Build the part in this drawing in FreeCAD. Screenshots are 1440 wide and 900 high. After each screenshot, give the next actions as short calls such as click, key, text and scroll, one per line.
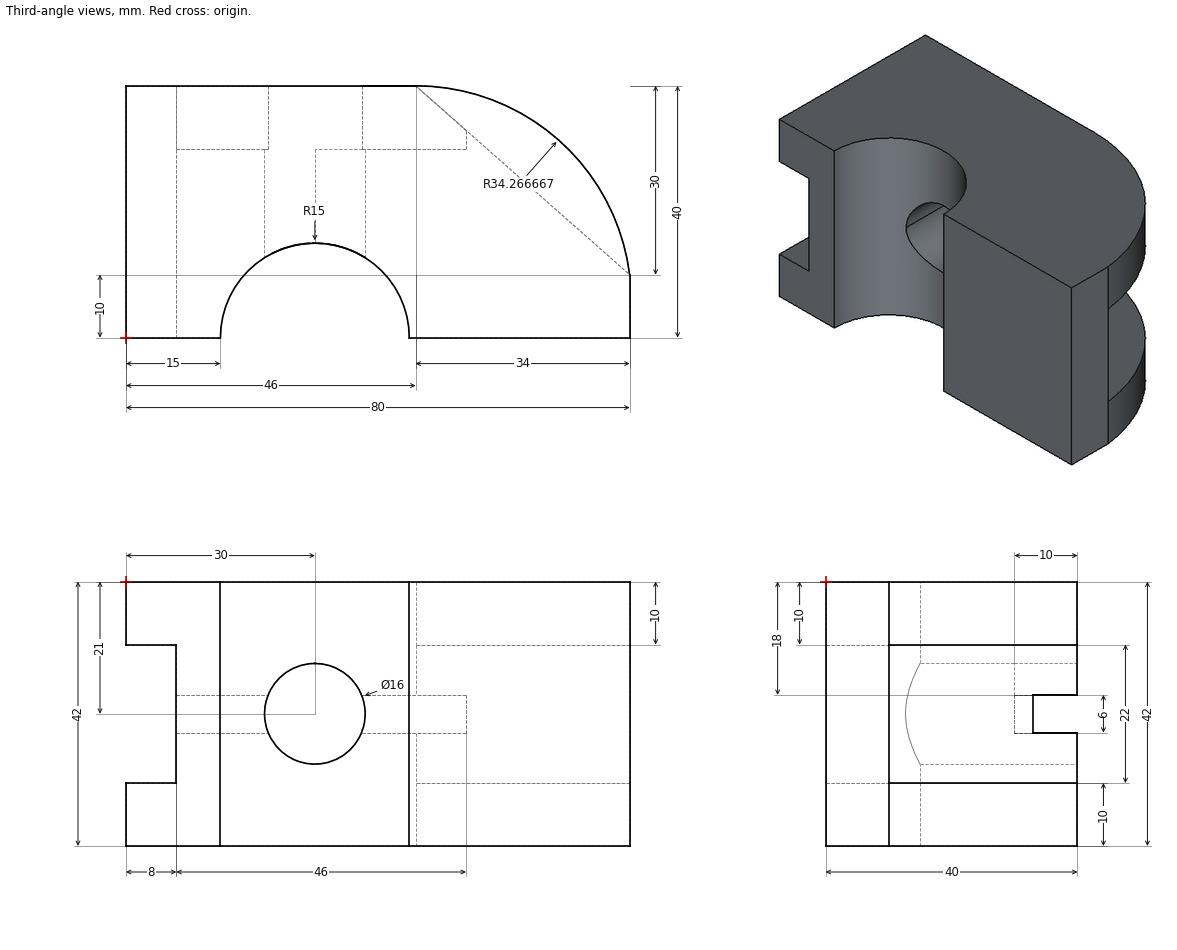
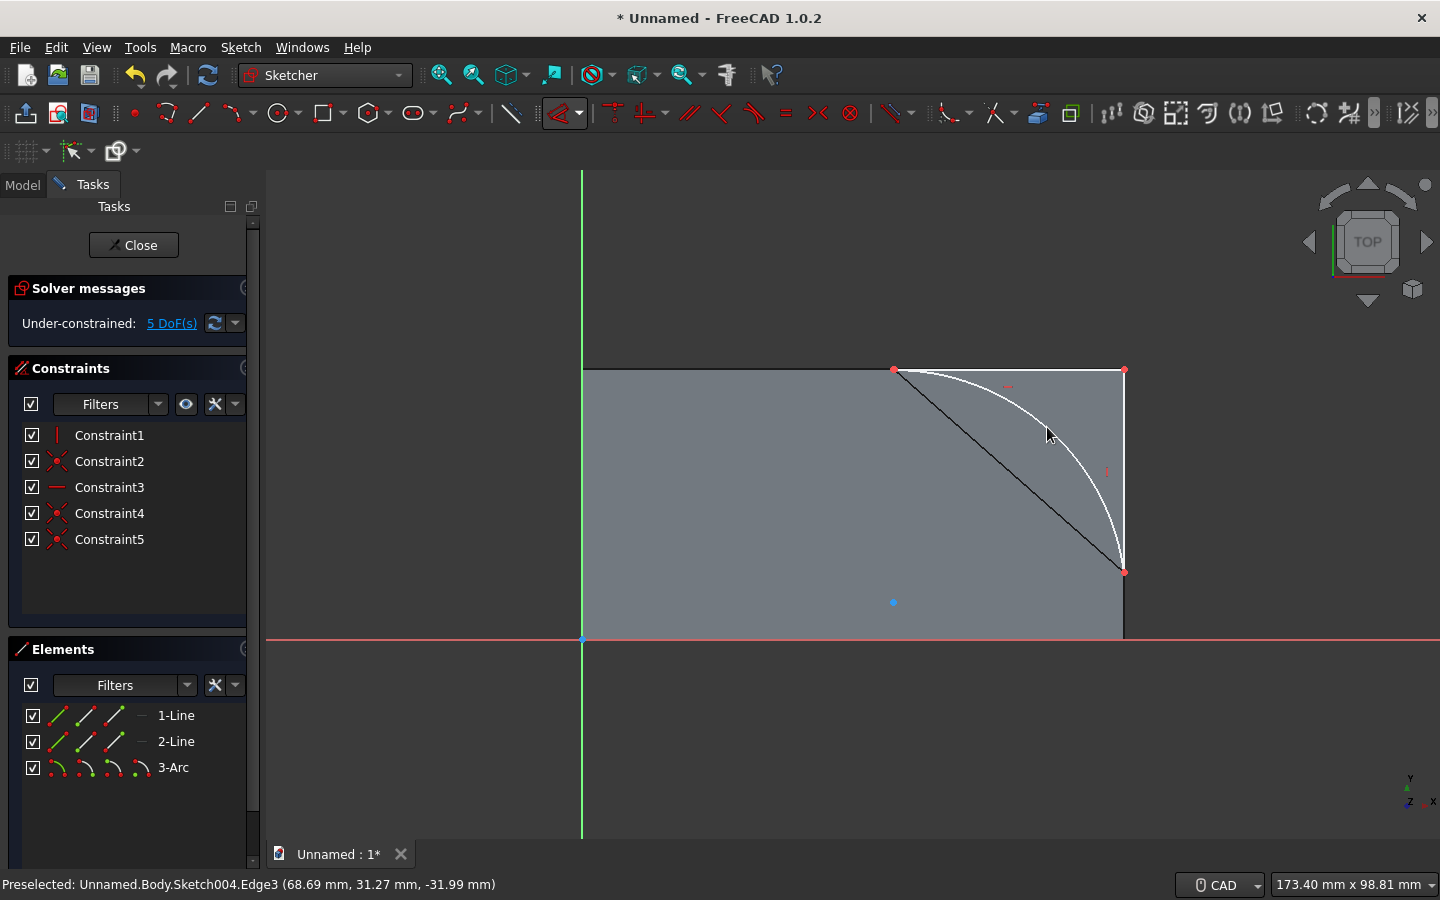
click(1055, 370)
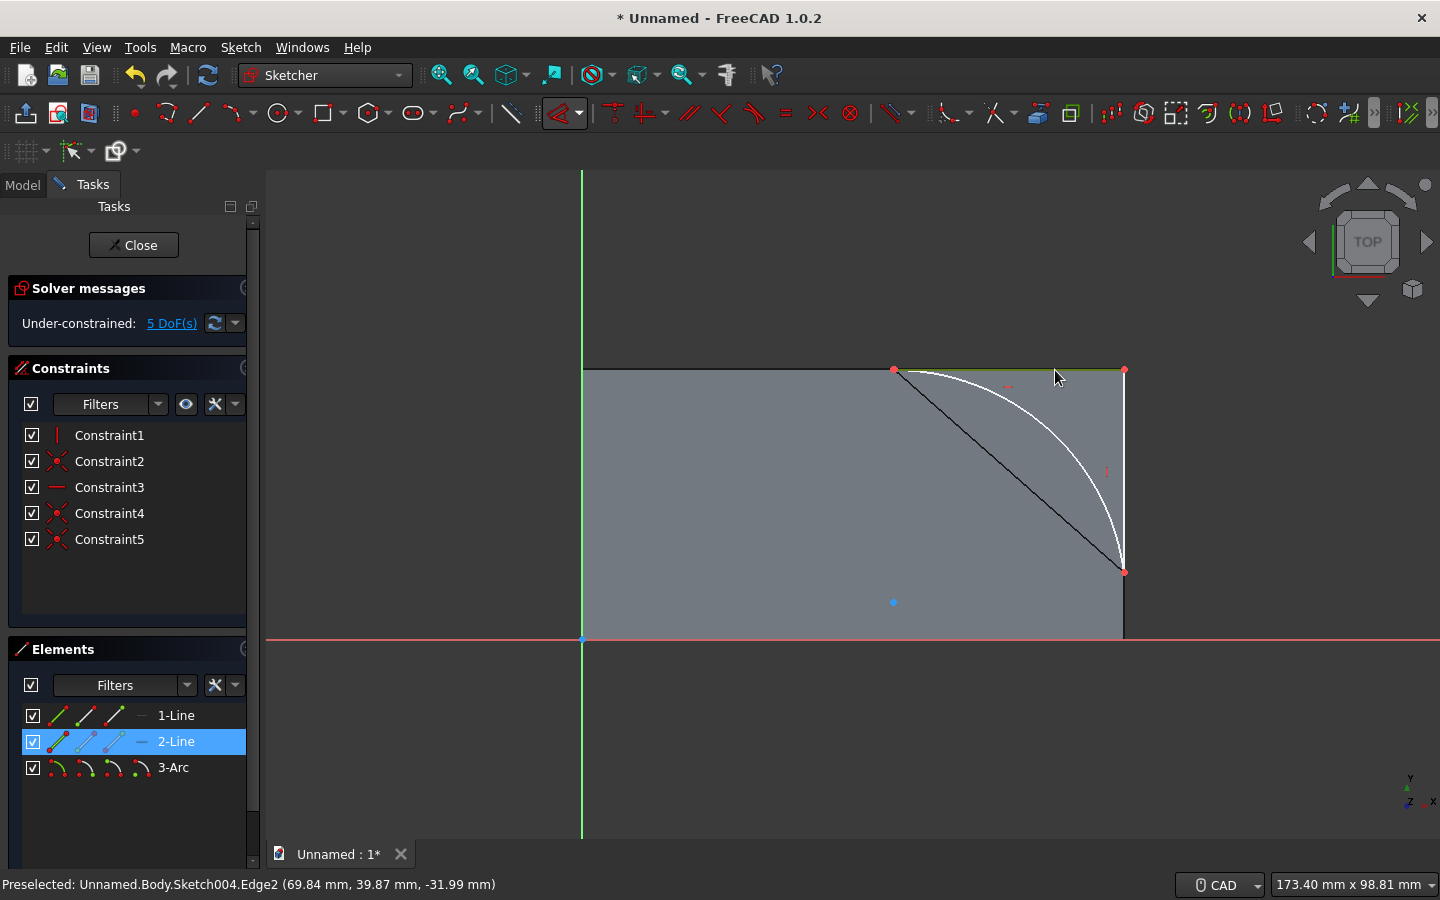
click(1090, 479)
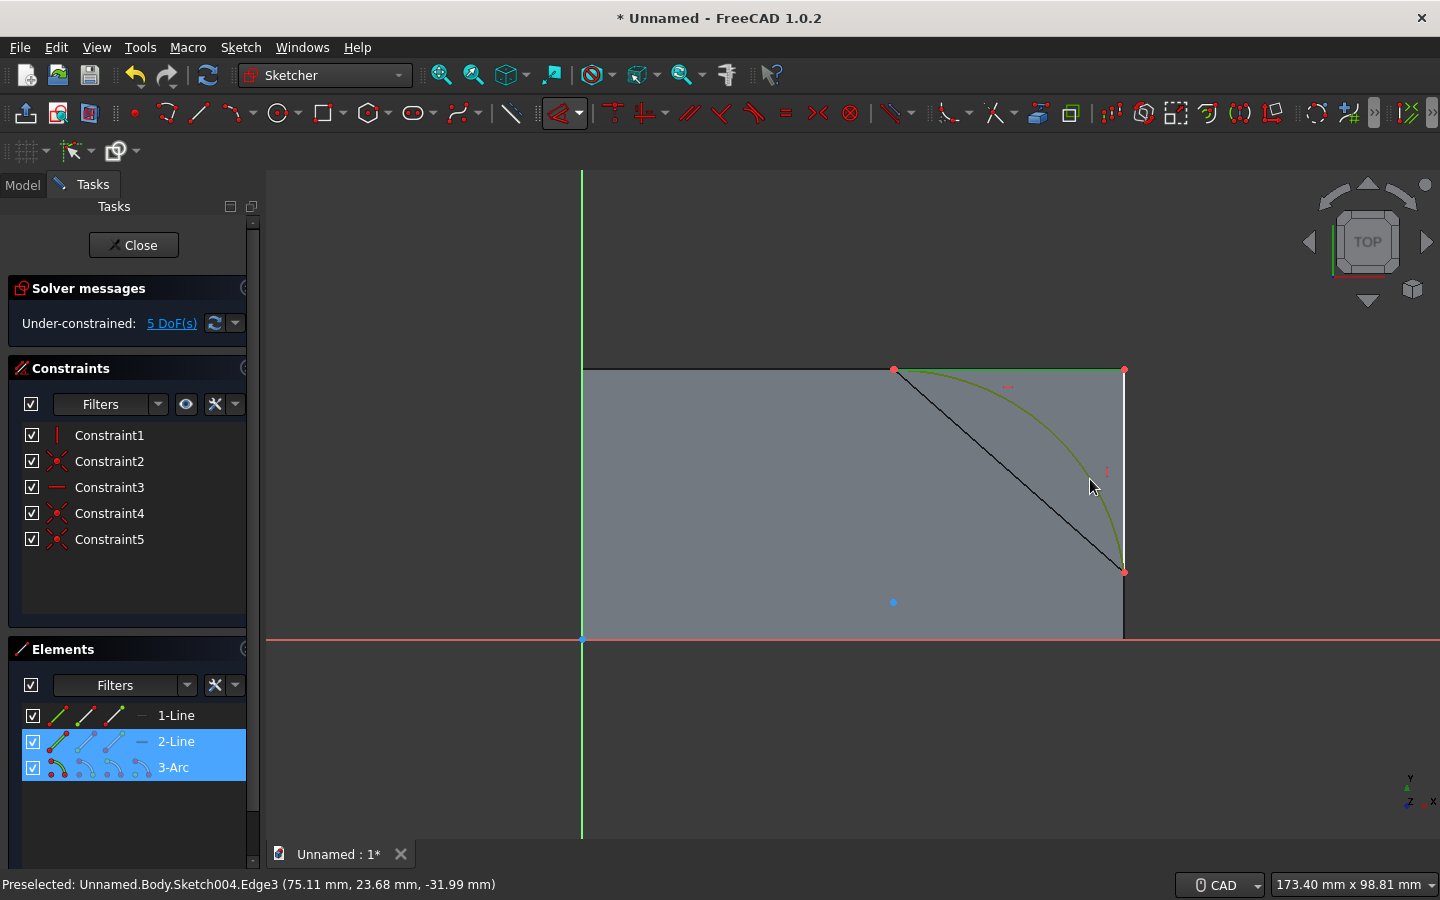
click(754, 114)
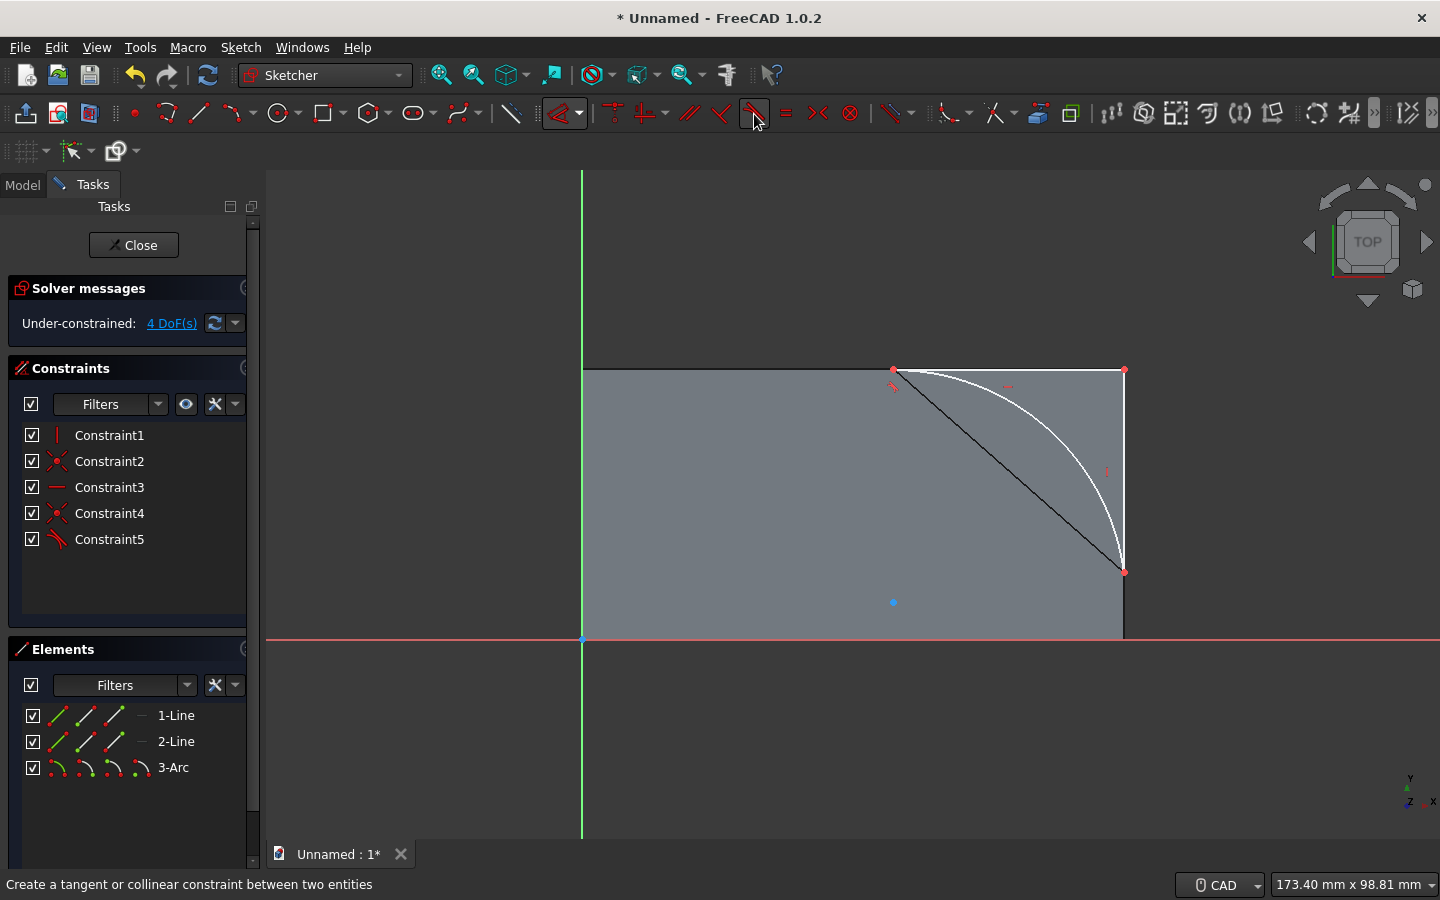
click(1090, 479)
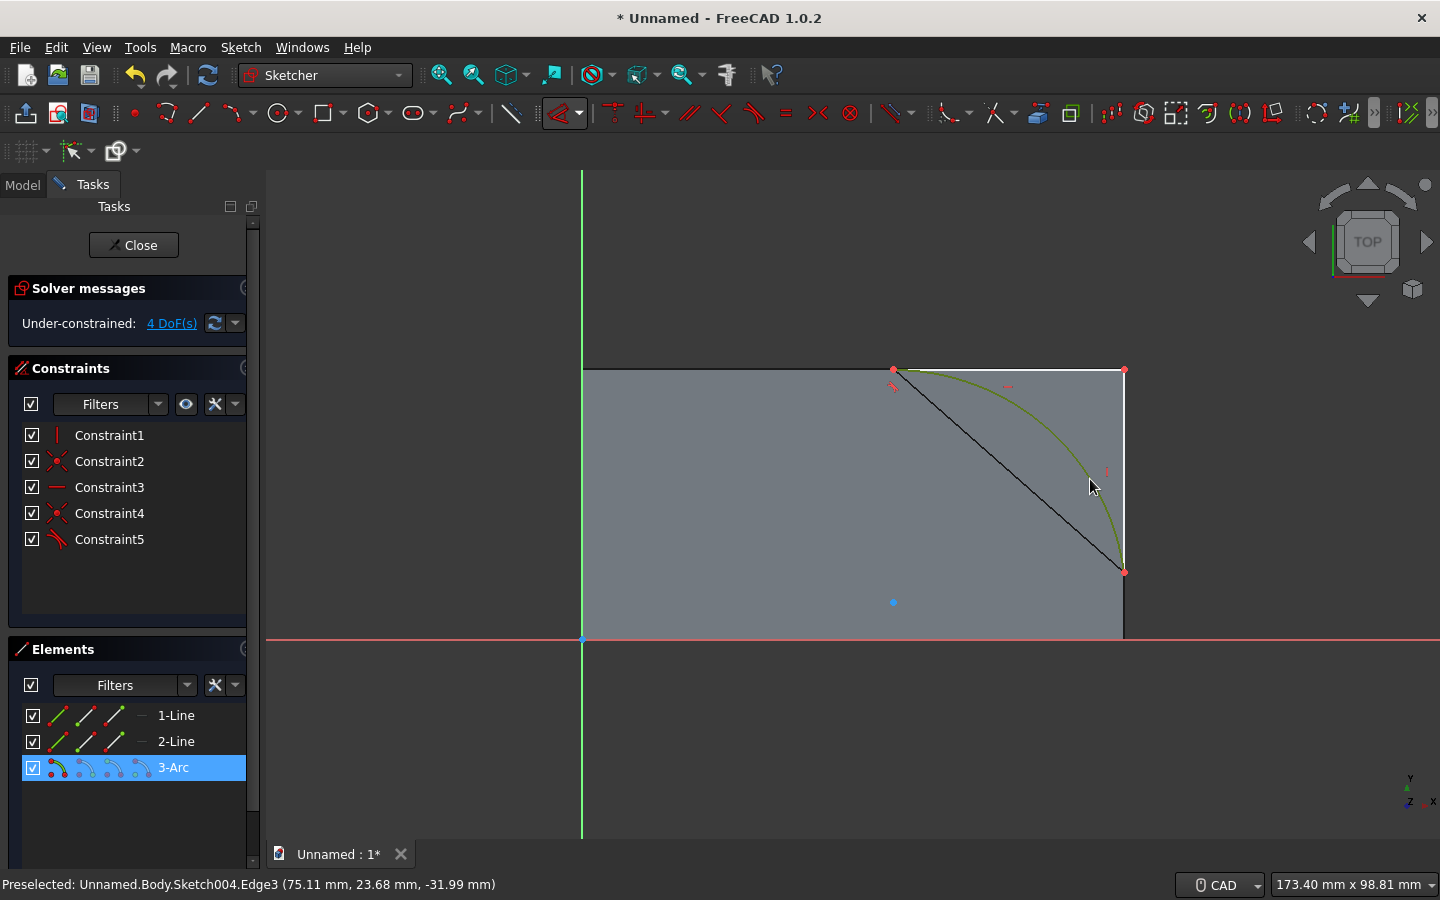
key(k)
key(r)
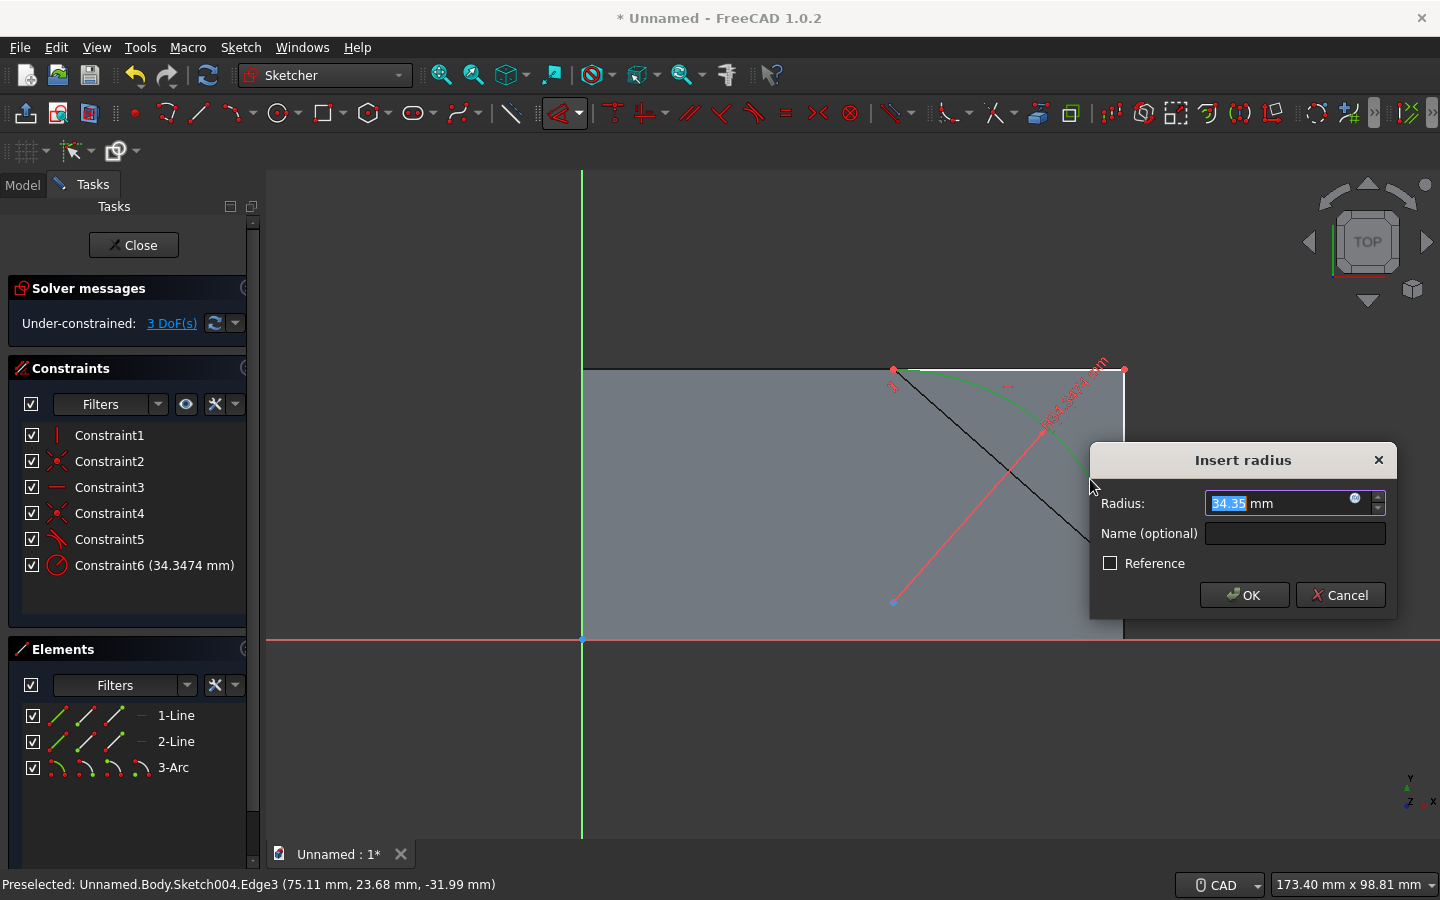
text(34.266667)
key(Return)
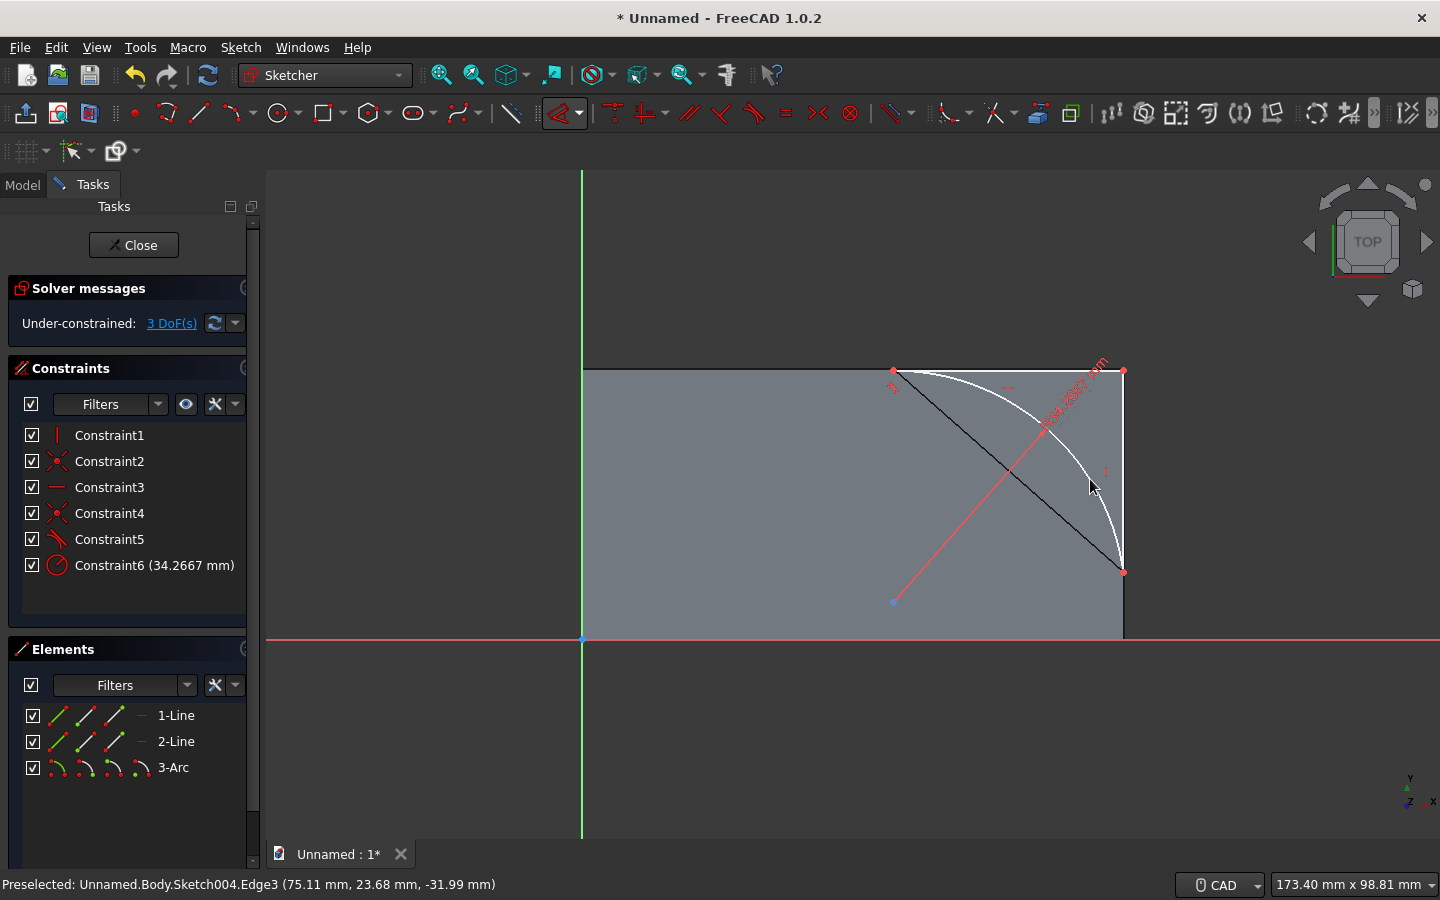
click(1123, 512)